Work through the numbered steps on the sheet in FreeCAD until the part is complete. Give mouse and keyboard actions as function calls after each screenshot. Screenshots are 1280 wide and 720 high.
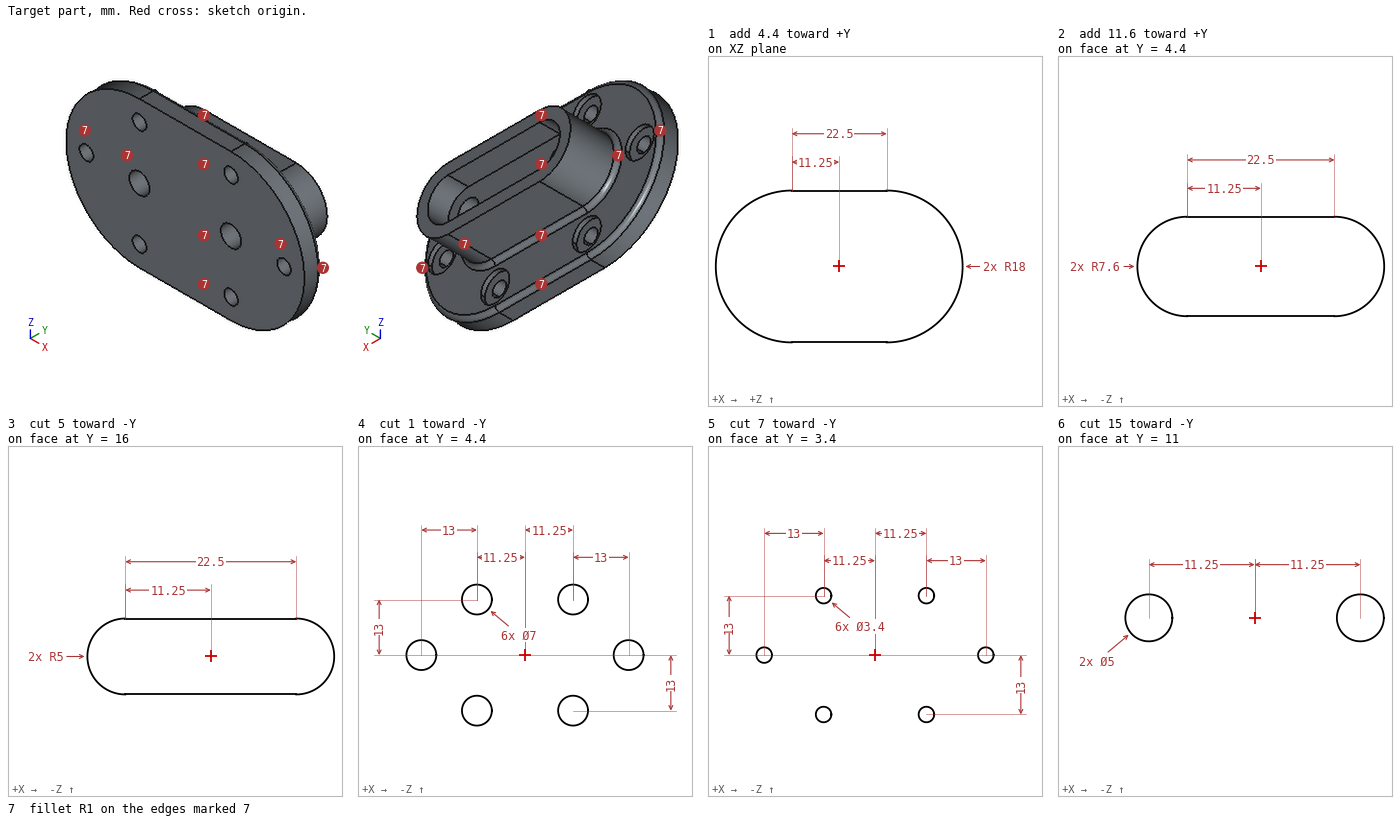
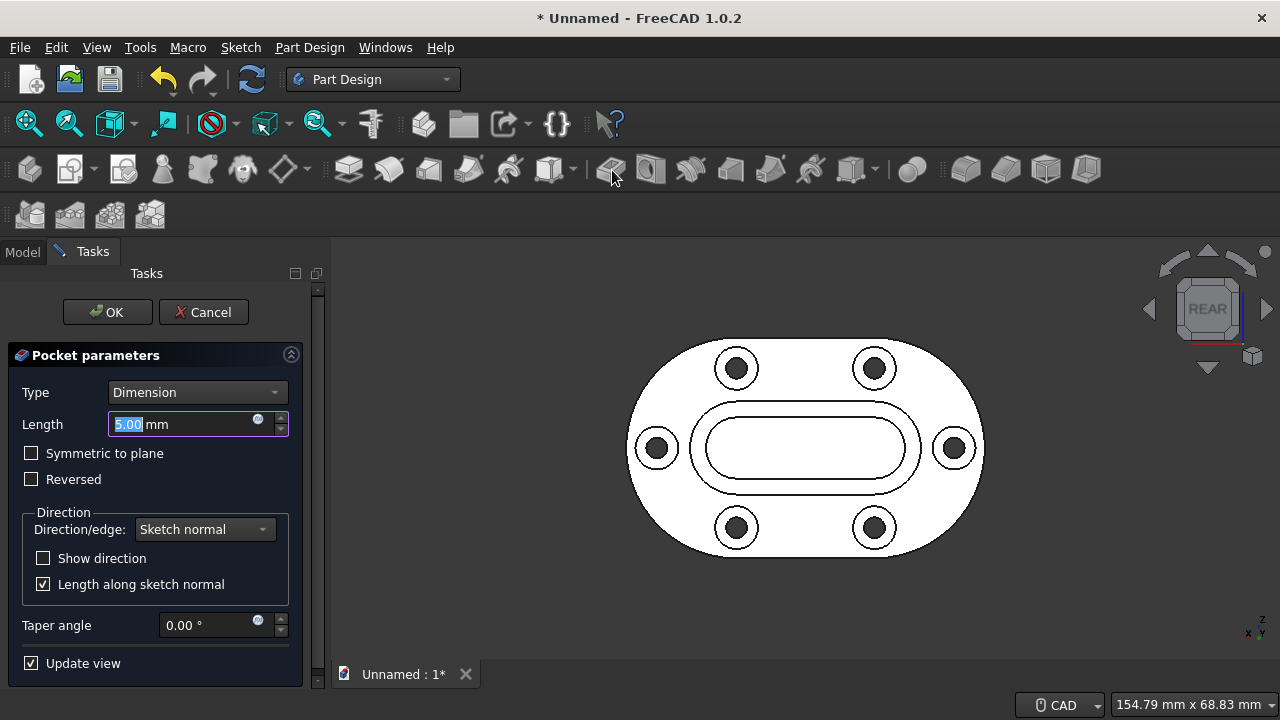
text(7)
key(Tab)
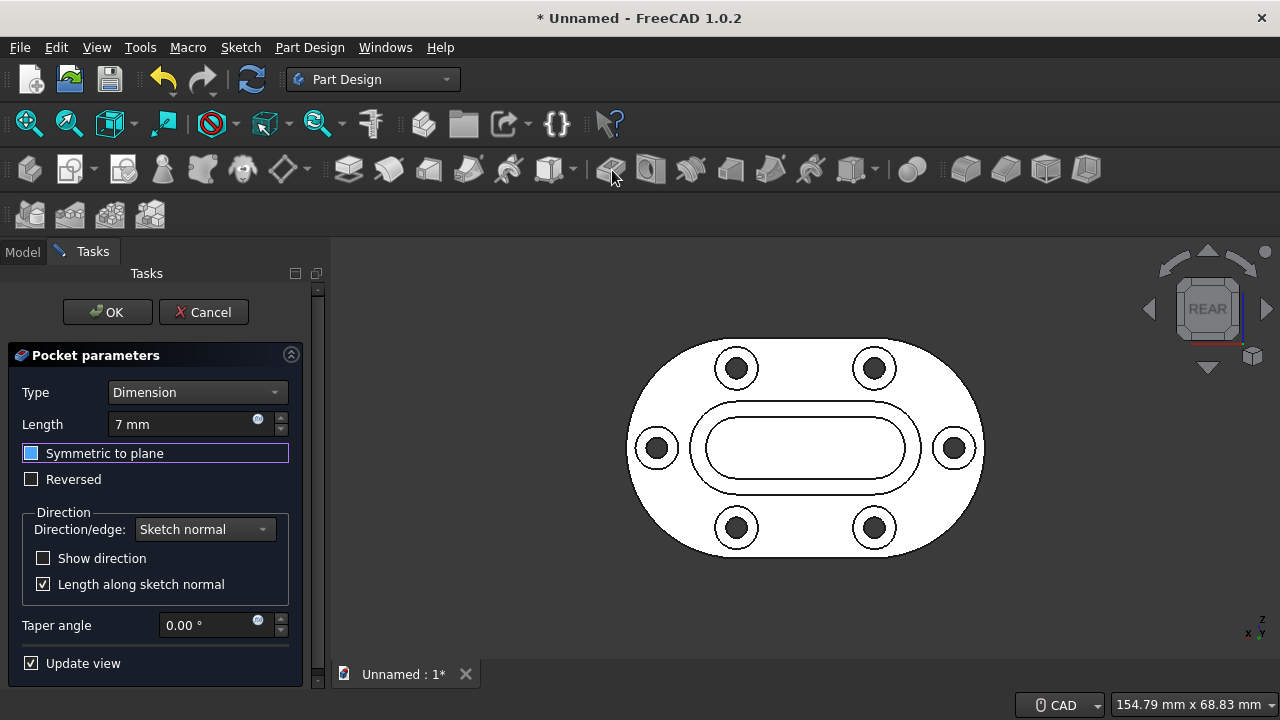
click(108, 312)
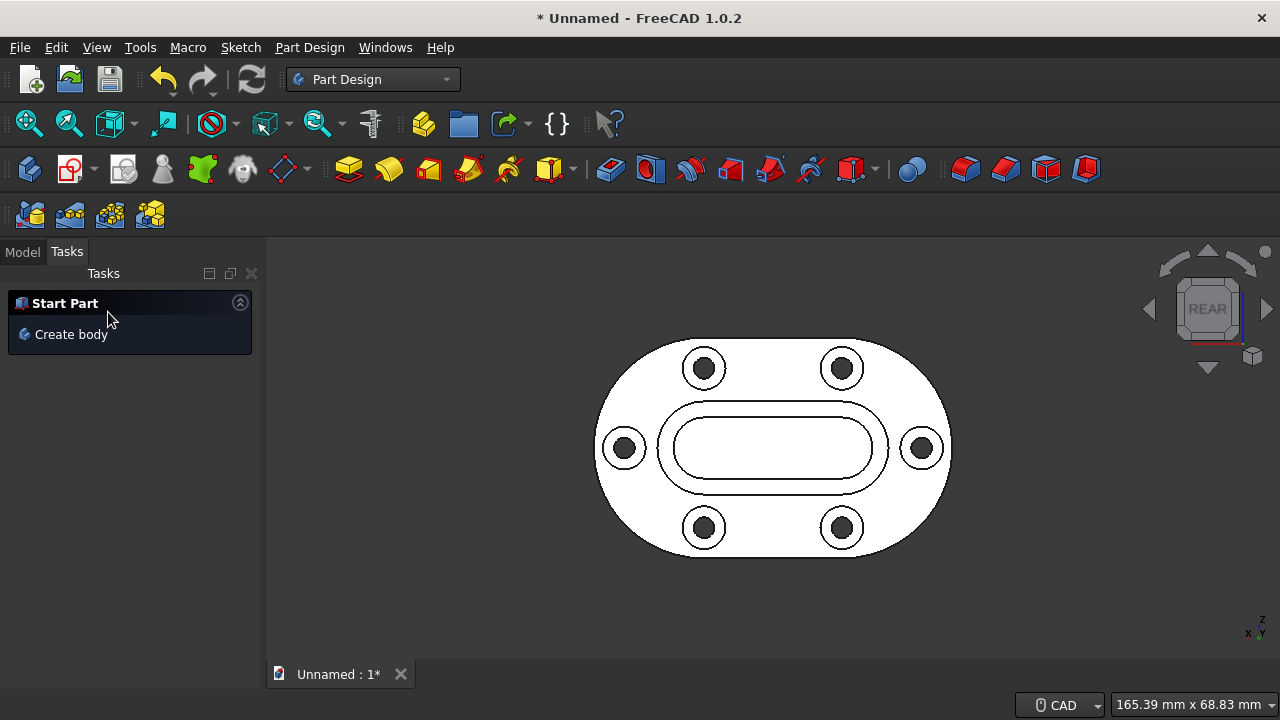
click(716, 447)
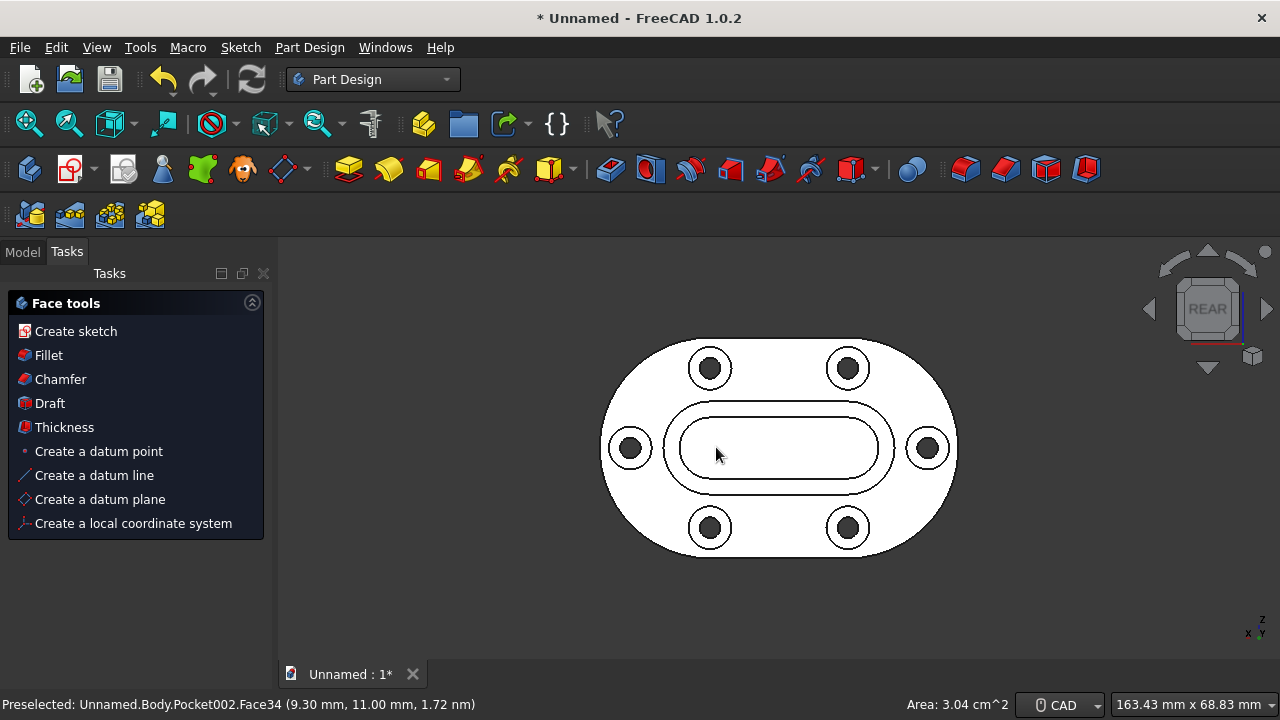
click(70, 170)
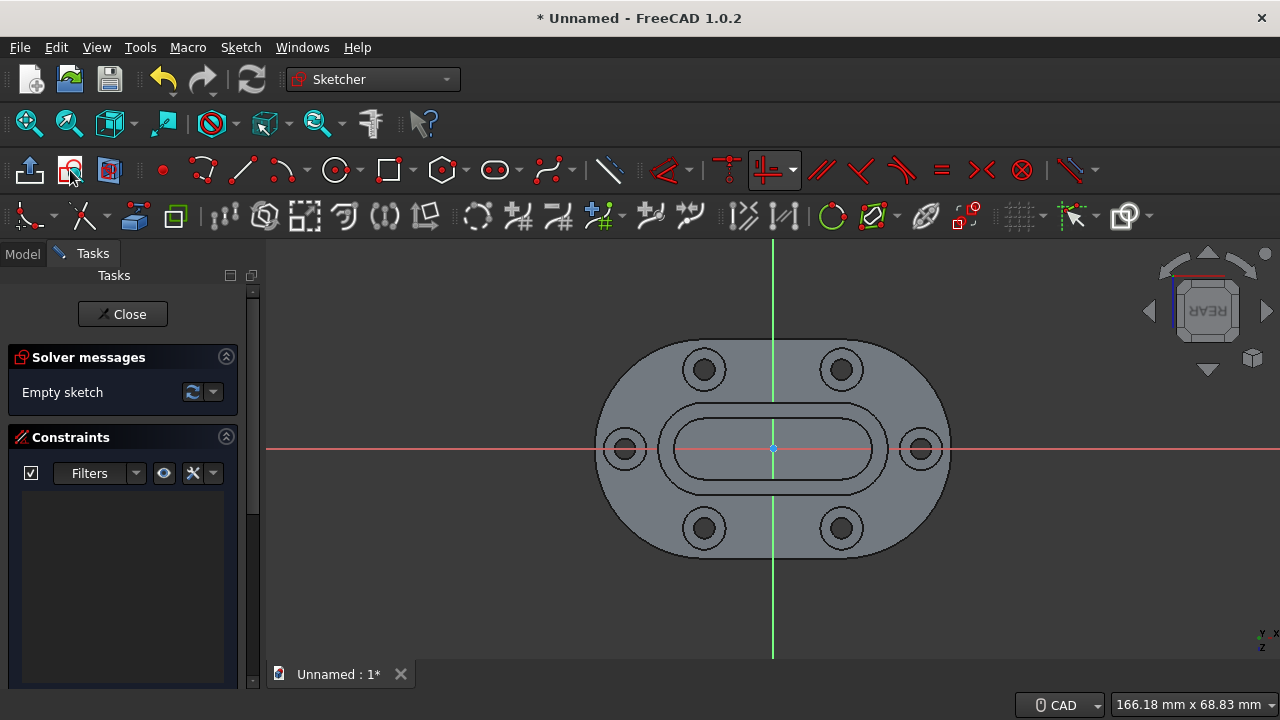
scroll(803, 449, up, 6)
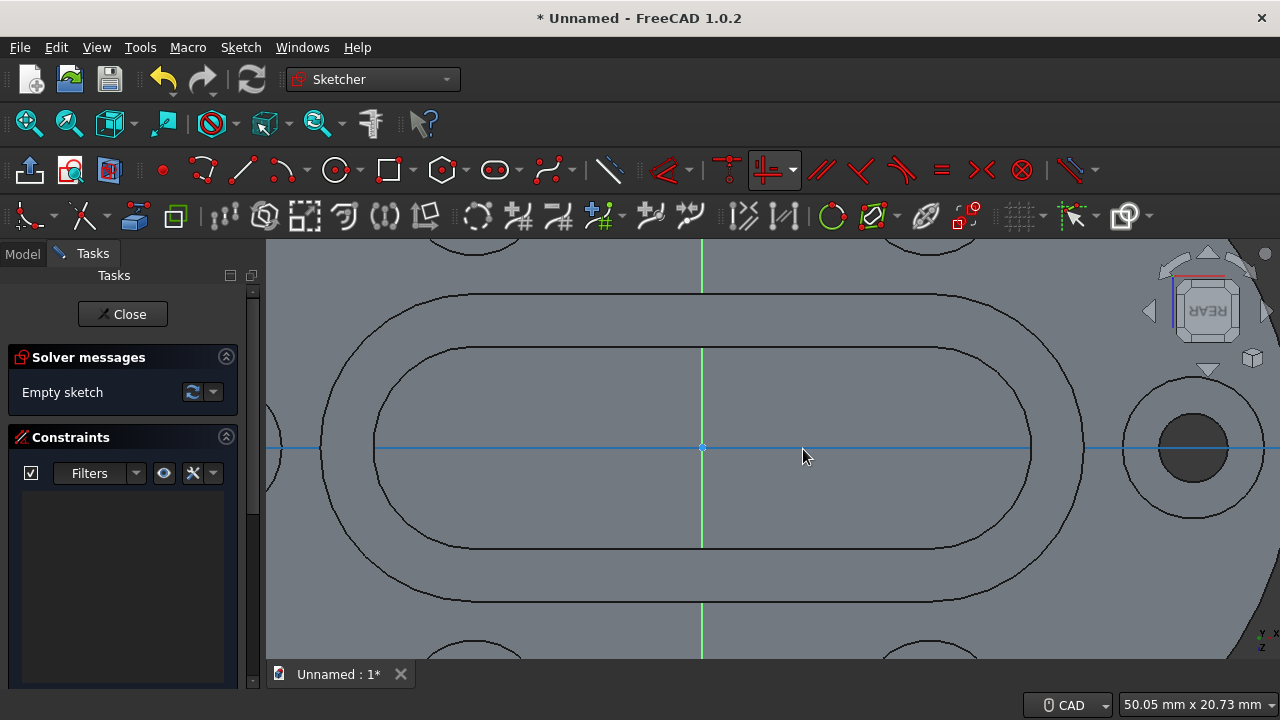
click(336, 170)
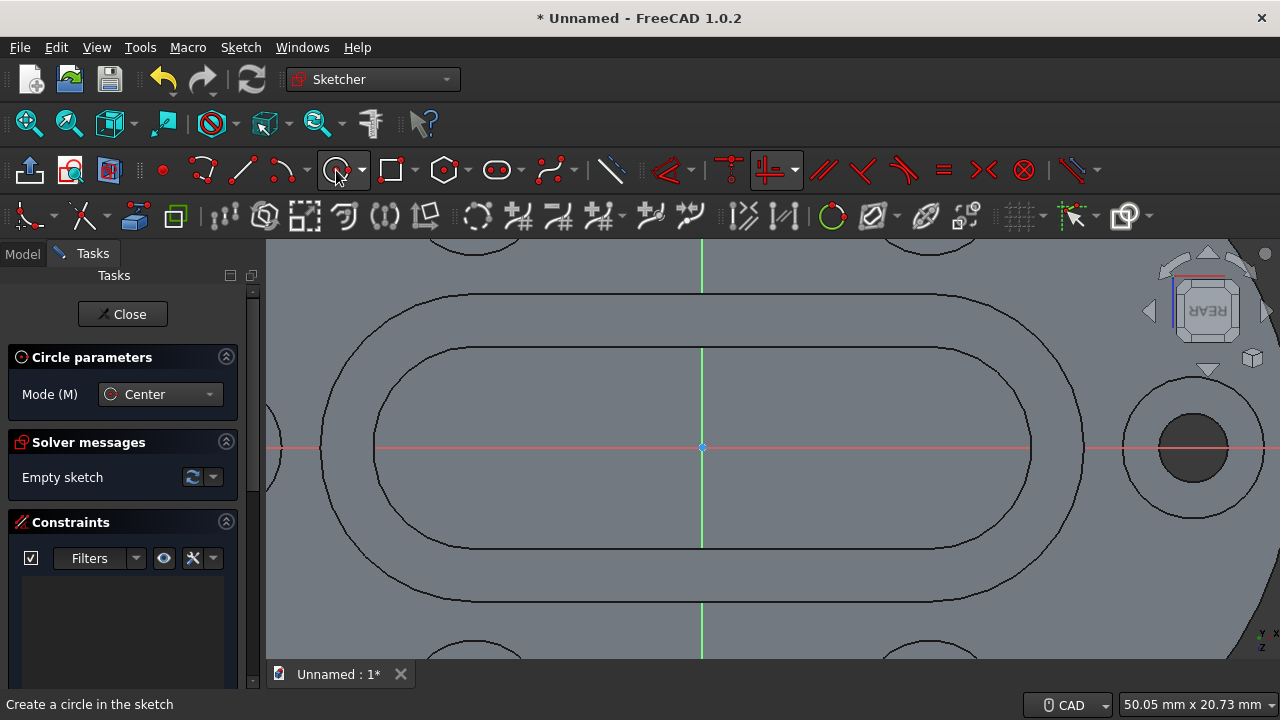
click(474, 448)
move(510, 412)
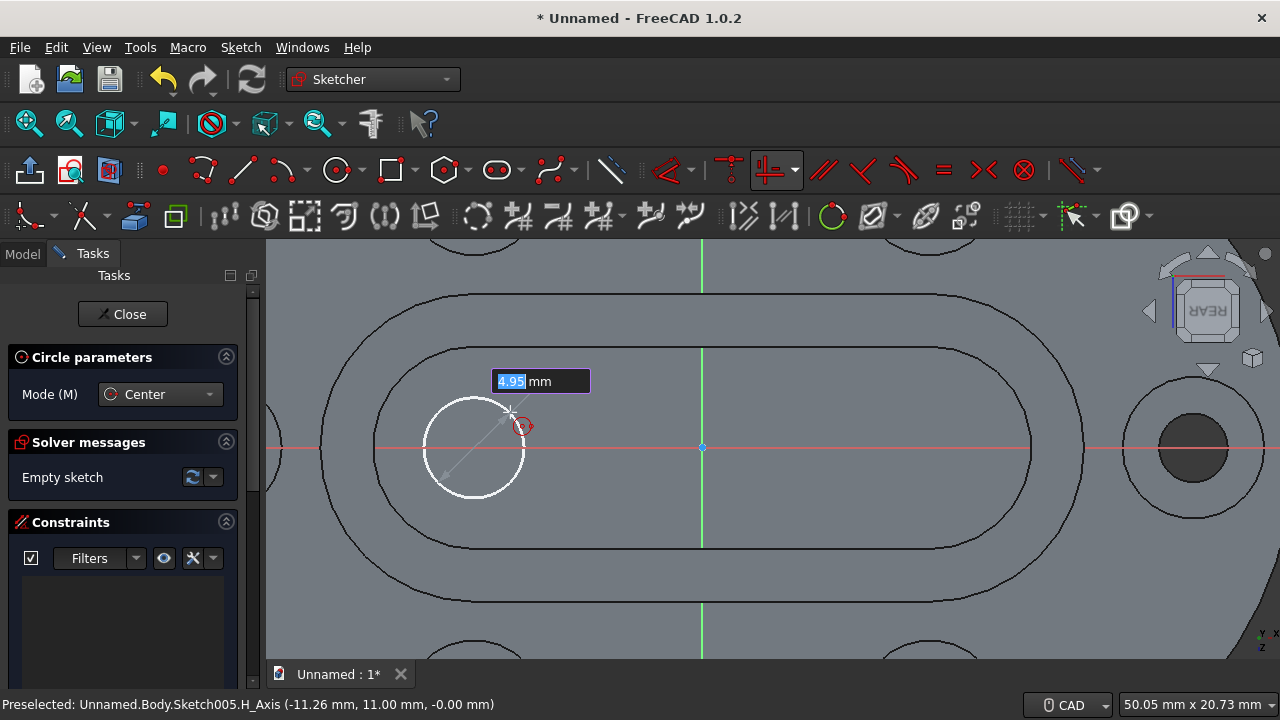
text(5)
key(Return)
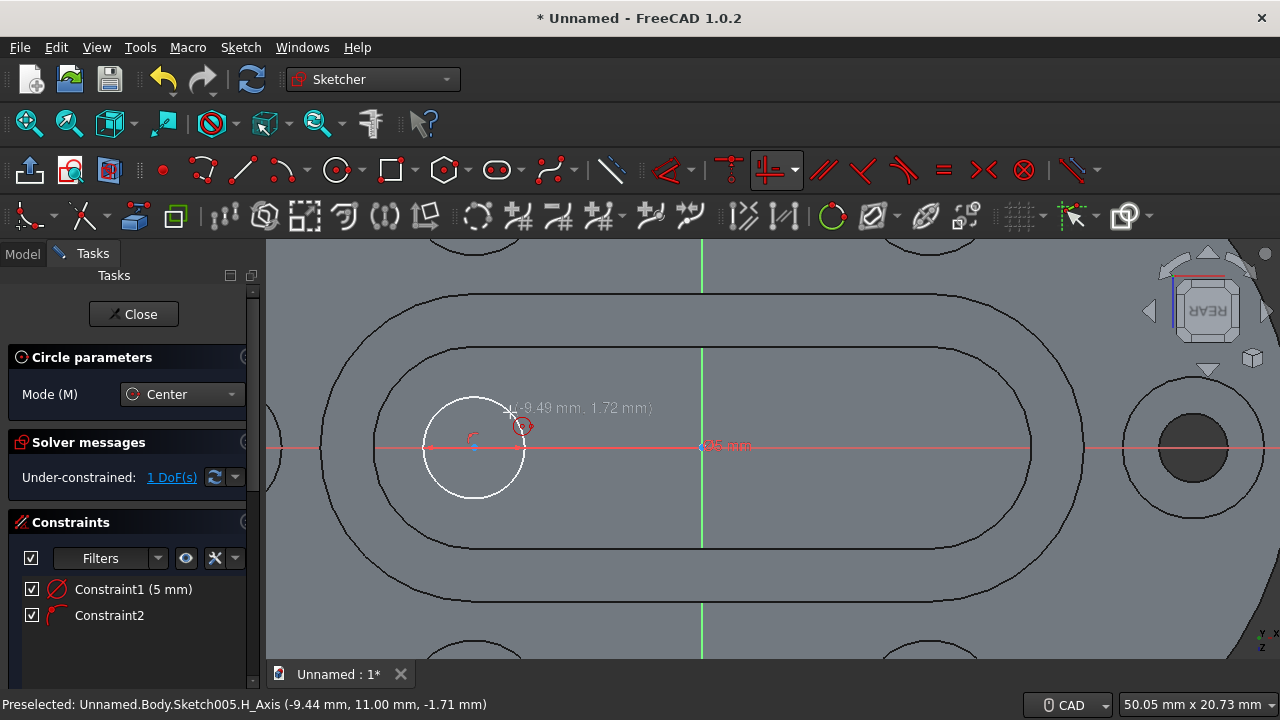
click(930, 448)
move(966, 412)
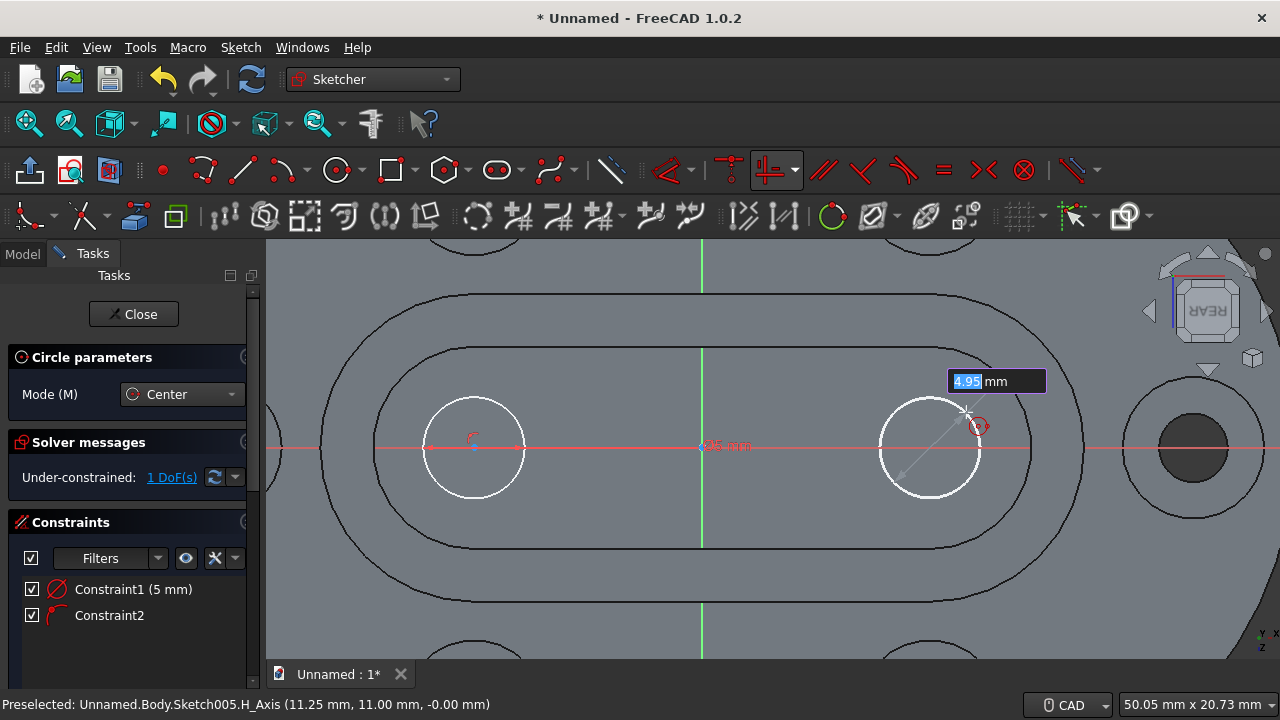
text(5)
key(Return)
key(Escape)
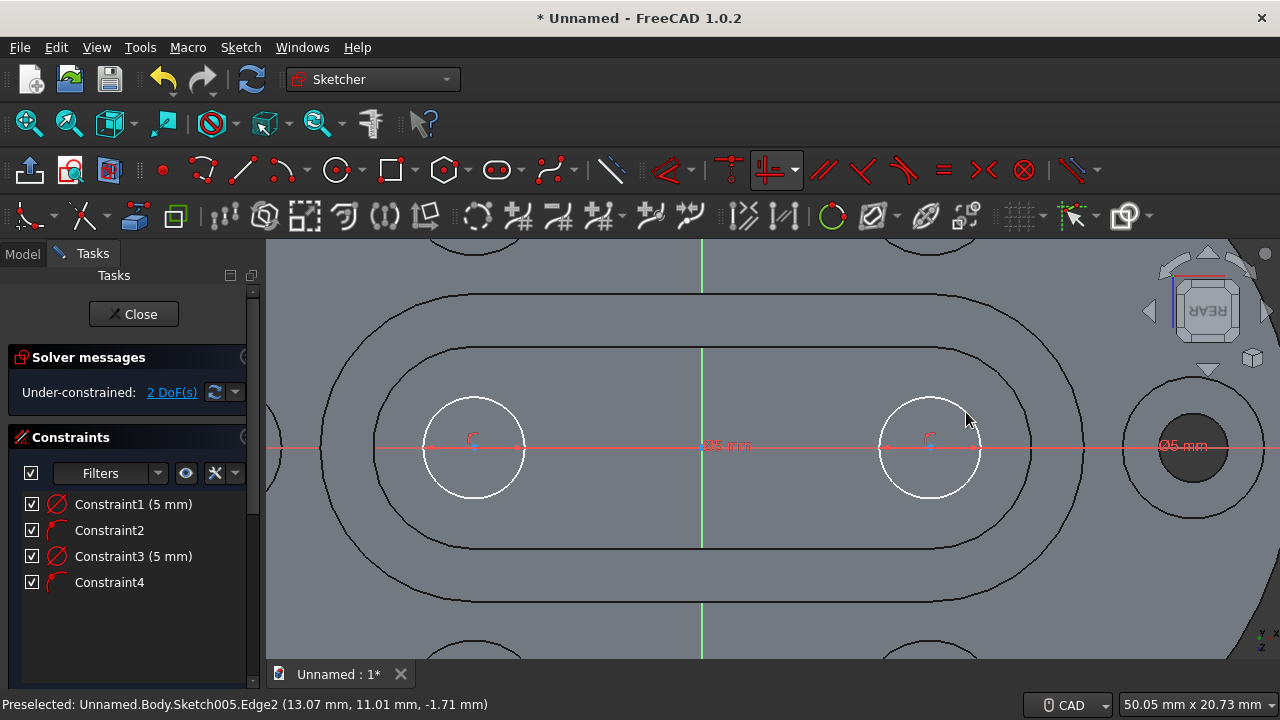
click(666, 170)